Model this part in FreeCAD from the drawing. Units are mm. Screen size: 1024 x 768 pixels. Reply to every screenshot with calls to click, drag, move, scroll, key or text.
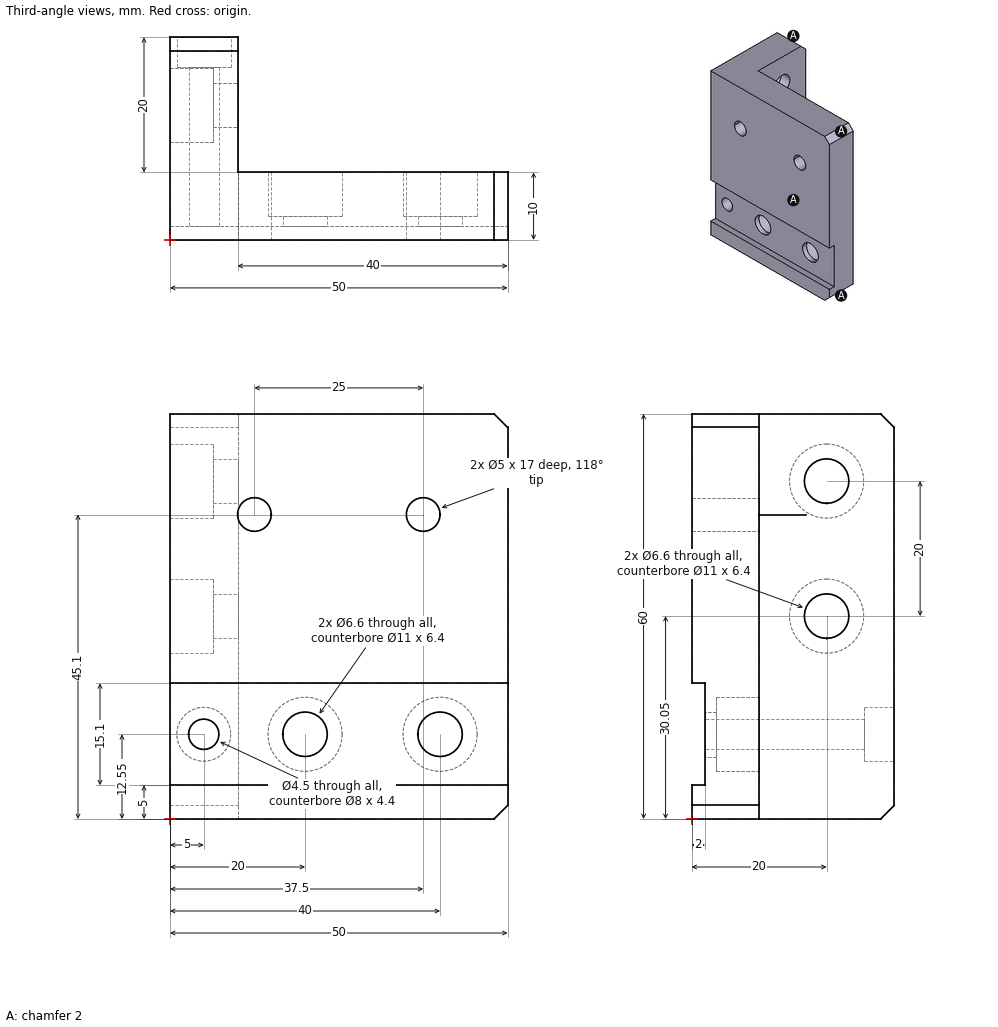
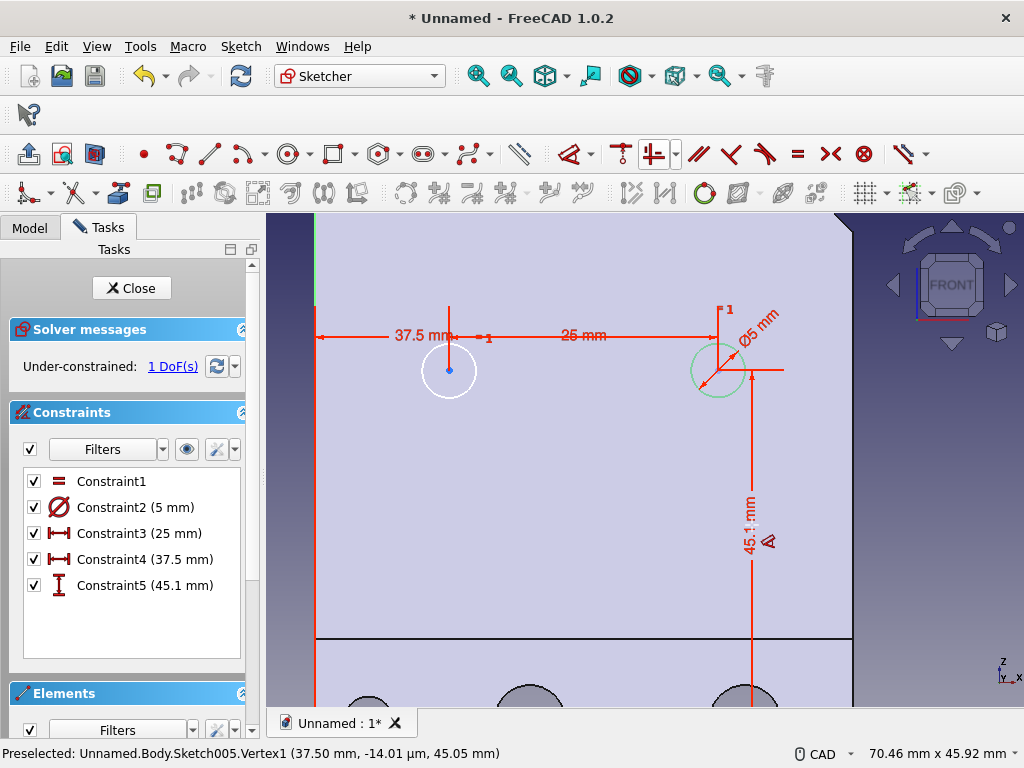
click(449, 371)
click(483, 525)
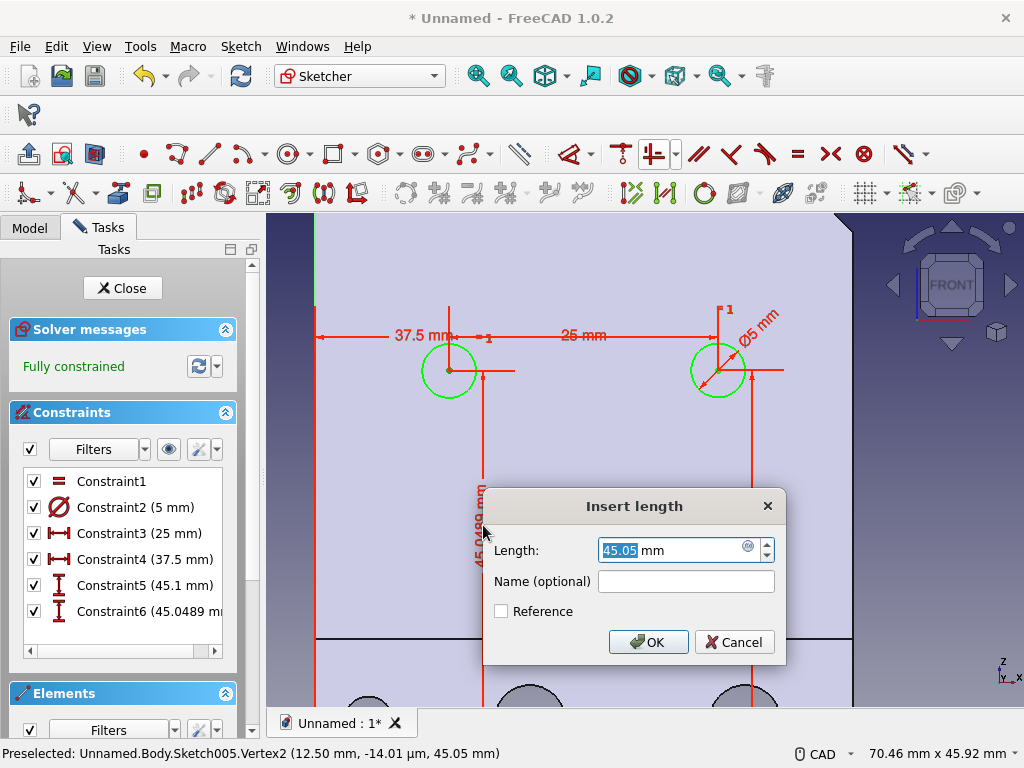
text(45.1)
key(Return)
key(Escape)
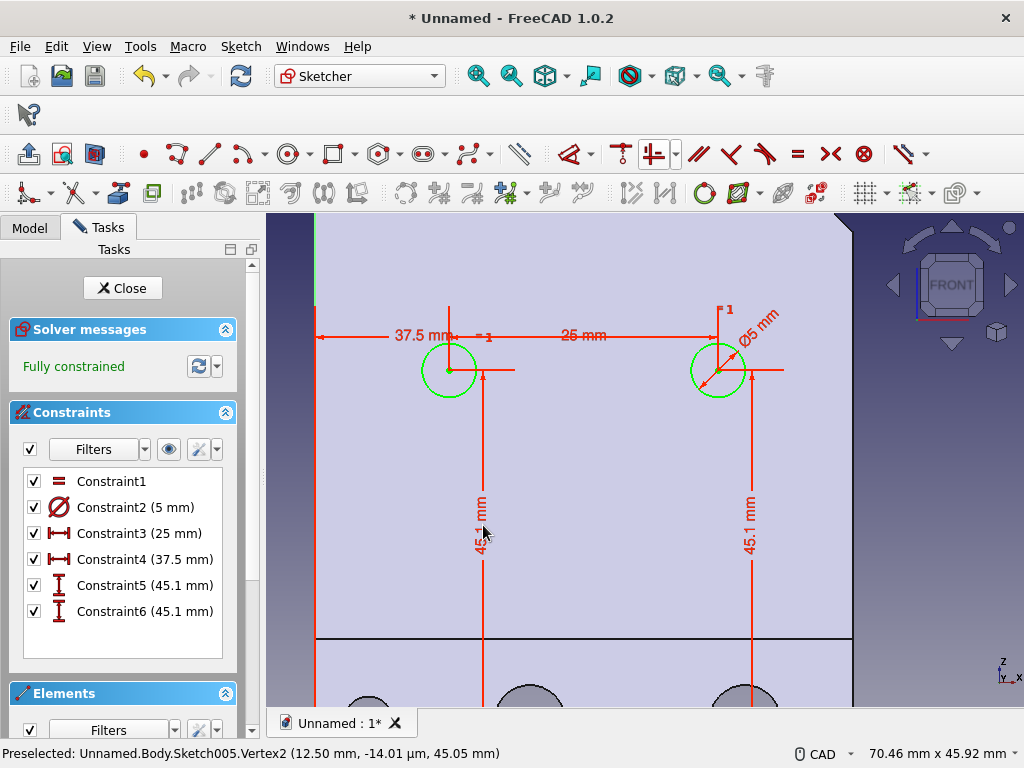
click(123, 288)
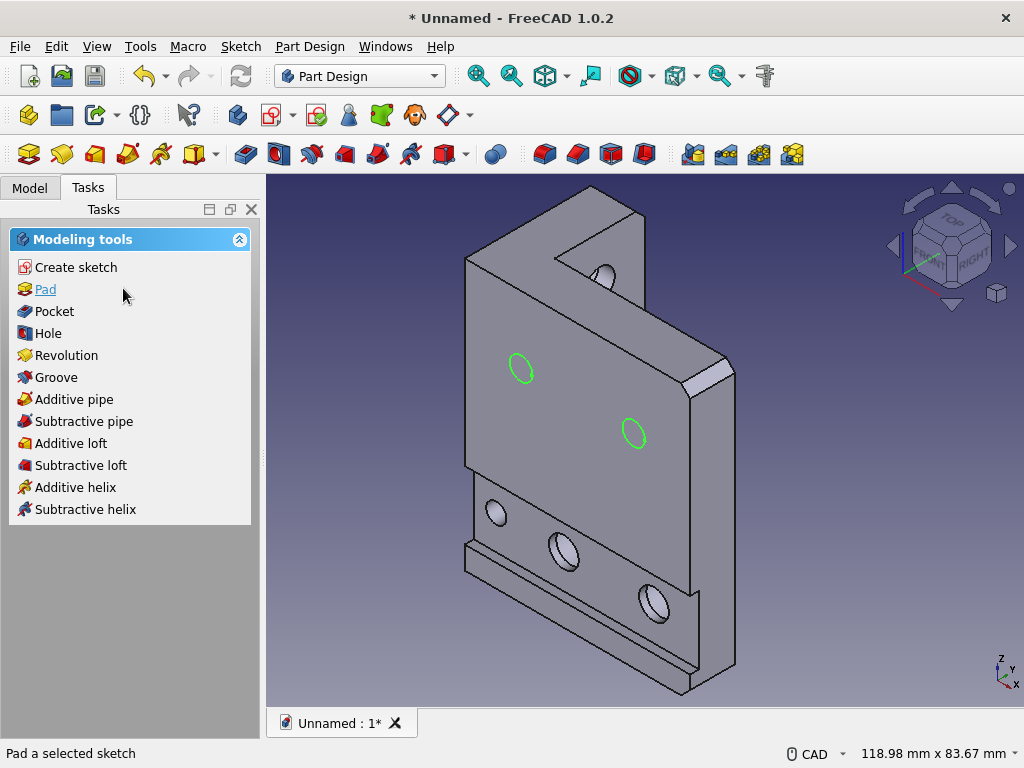
click(279, 154)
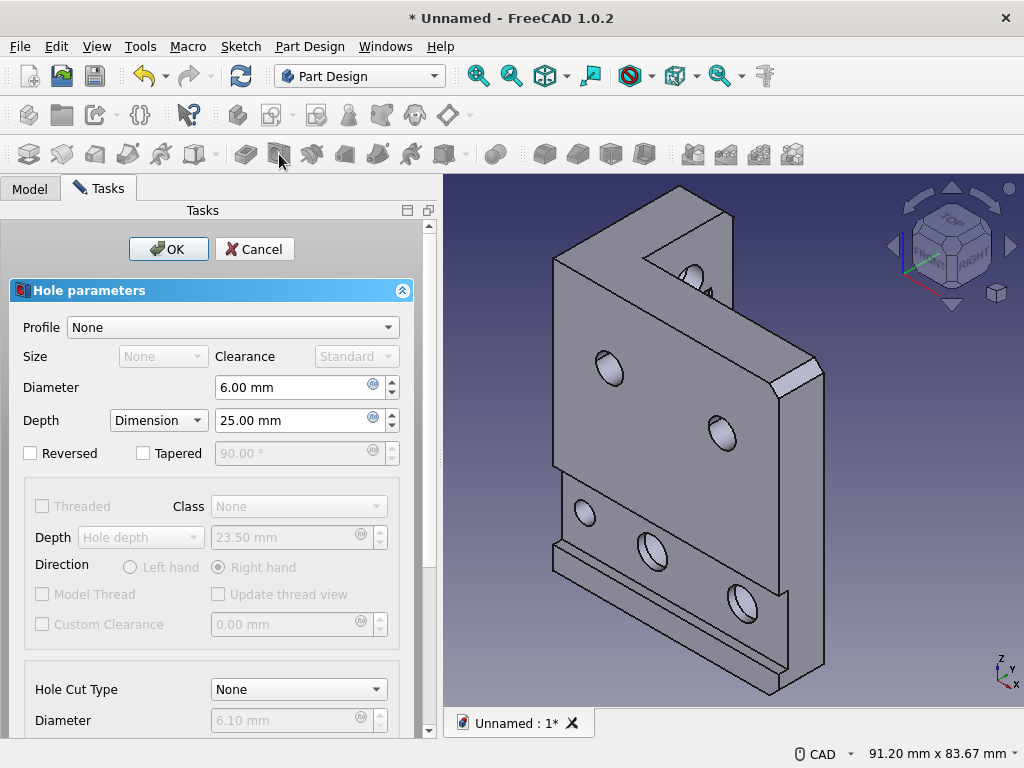
triple_click(300, 388)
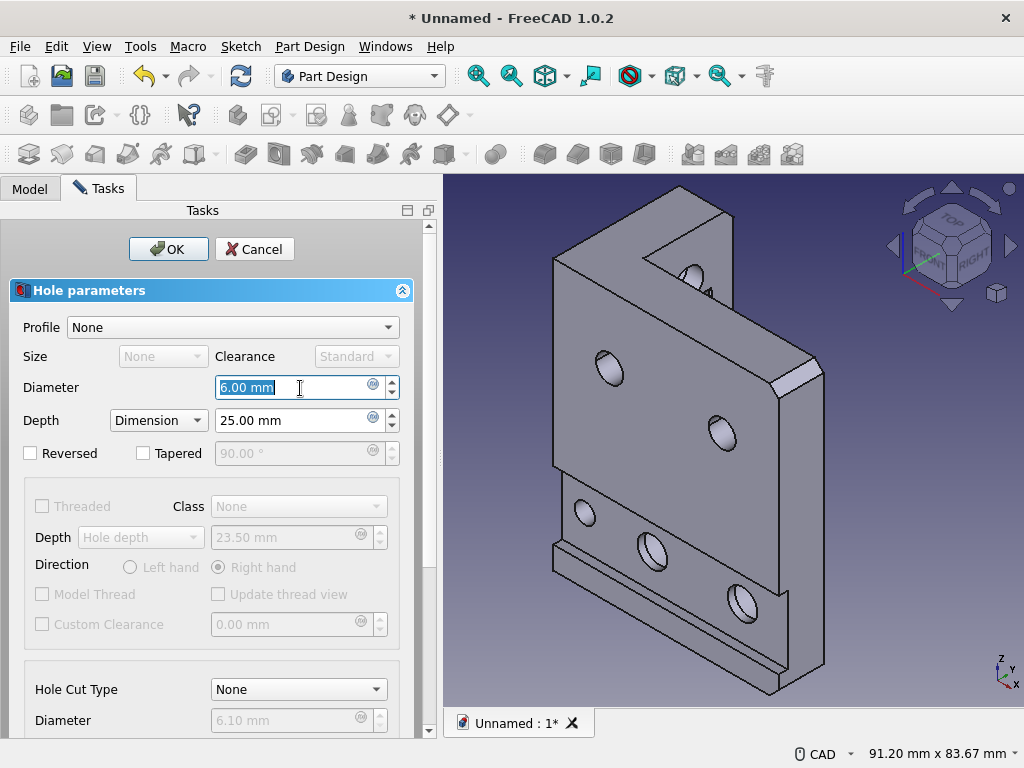
text(5)
key(Tab)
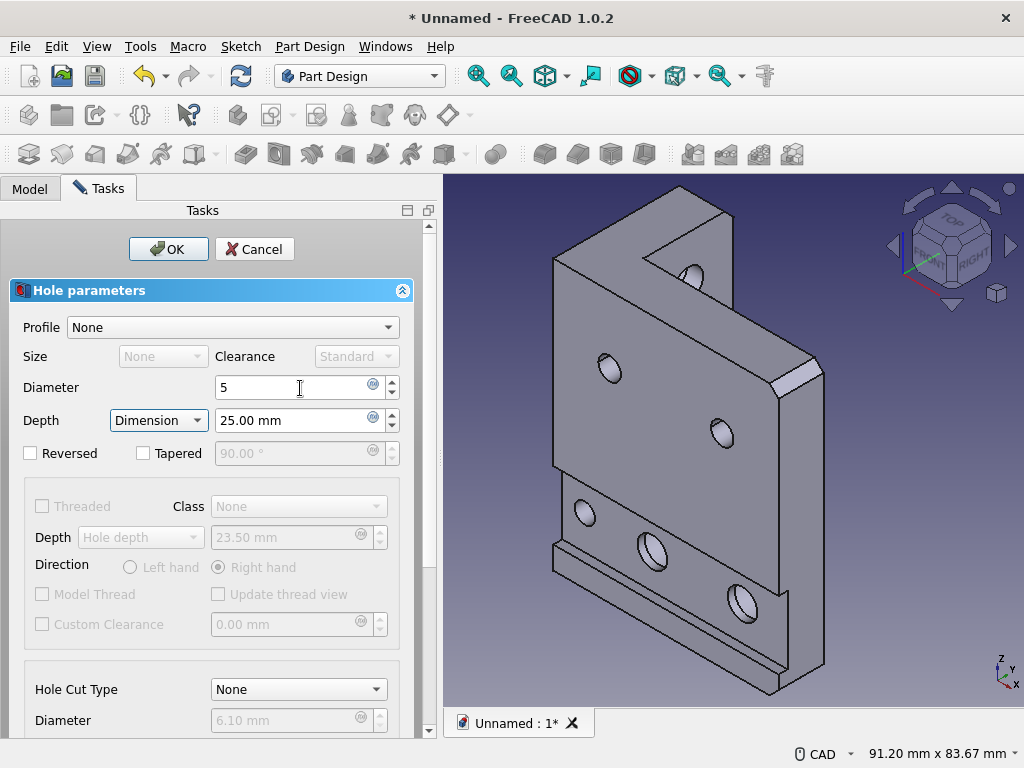
triple_click(300, 420)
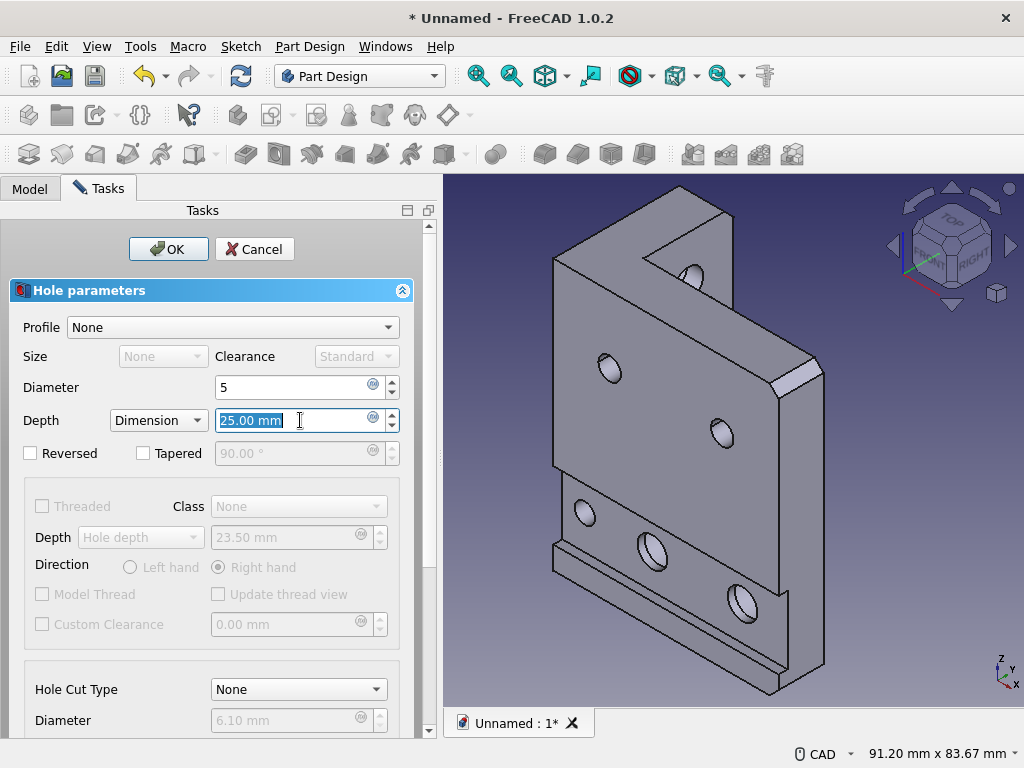
text(17)
key(Tab)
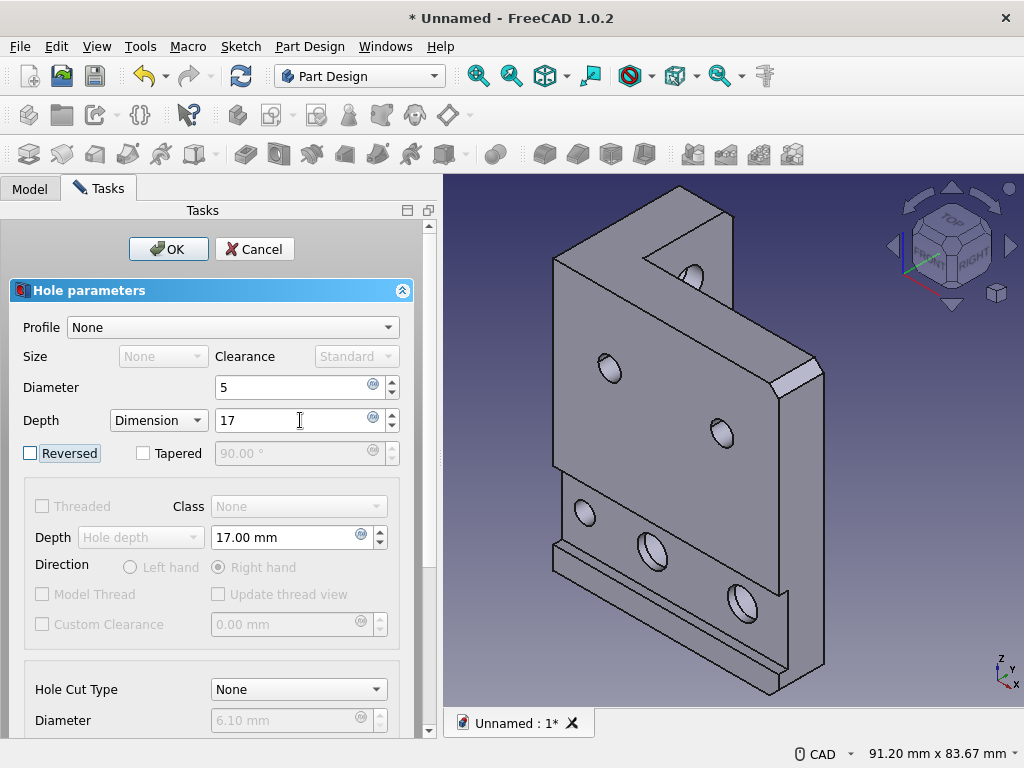
click(169, 249)